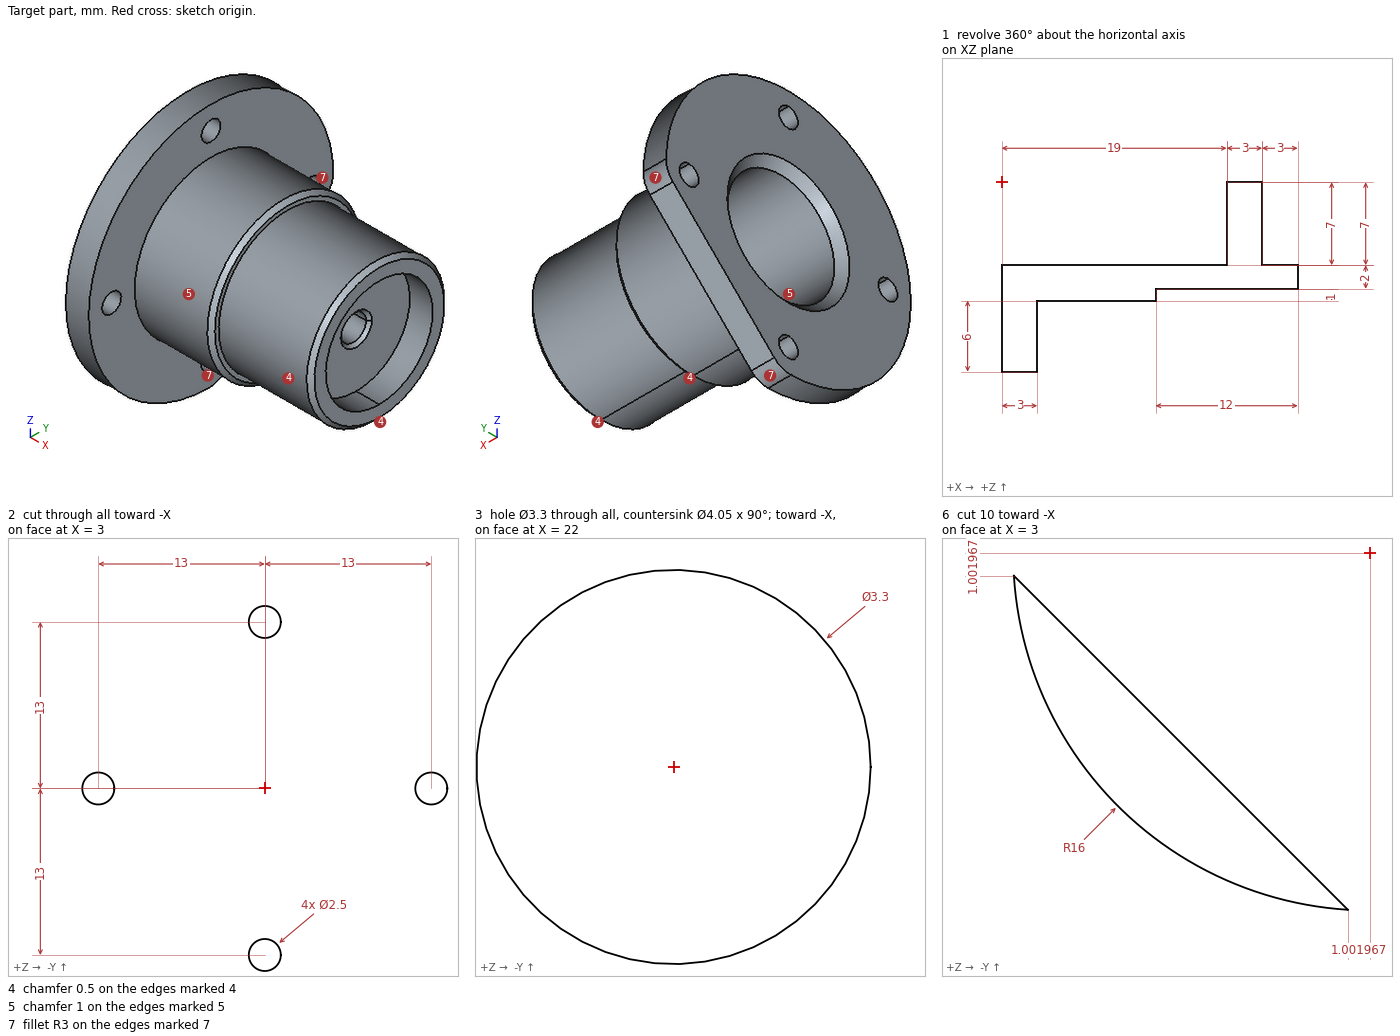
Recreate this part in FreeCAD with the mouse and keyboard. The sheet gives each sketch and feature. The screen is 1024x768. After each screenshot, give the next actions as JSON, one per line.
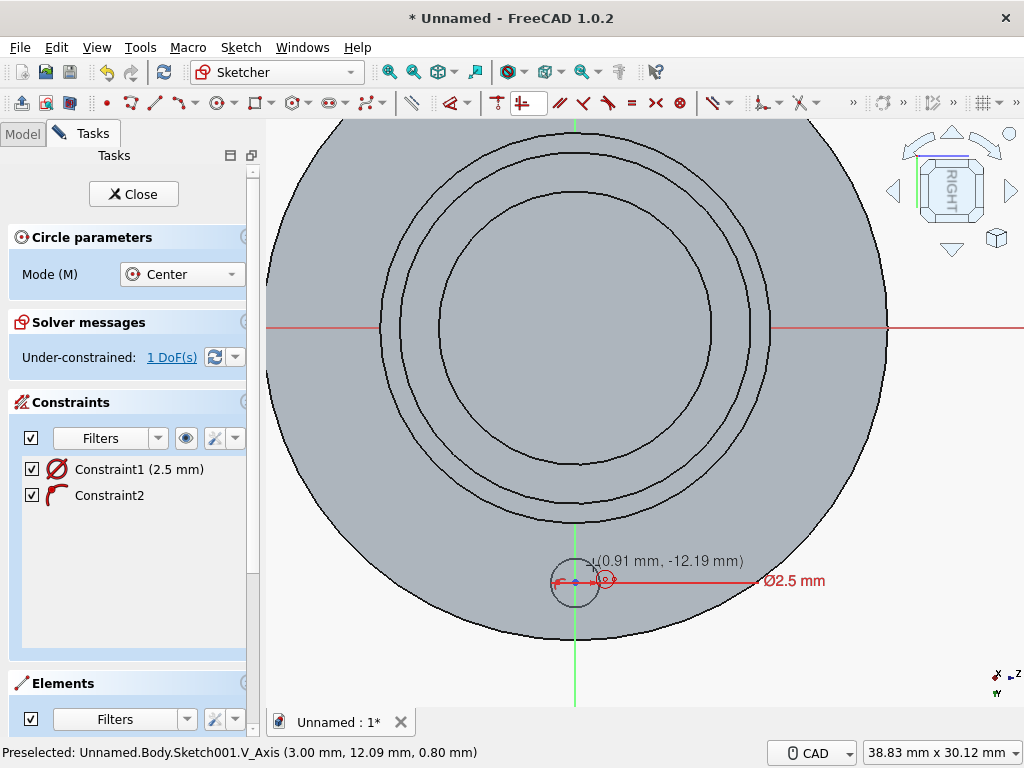
{"action": "left_click", "coordinate": [322, 328]}
{"action": "mouse_move", "coordinate": [339, 311]}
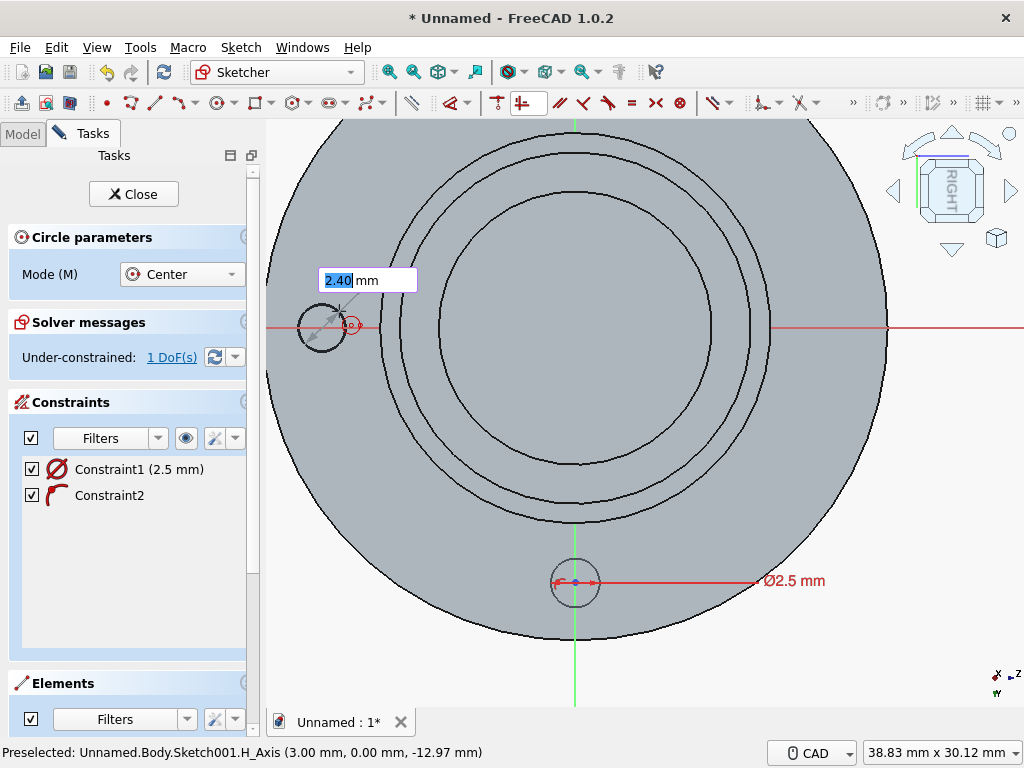
{"action": "type", "text": "2.5"}
{"action": "key", "text": "Return"}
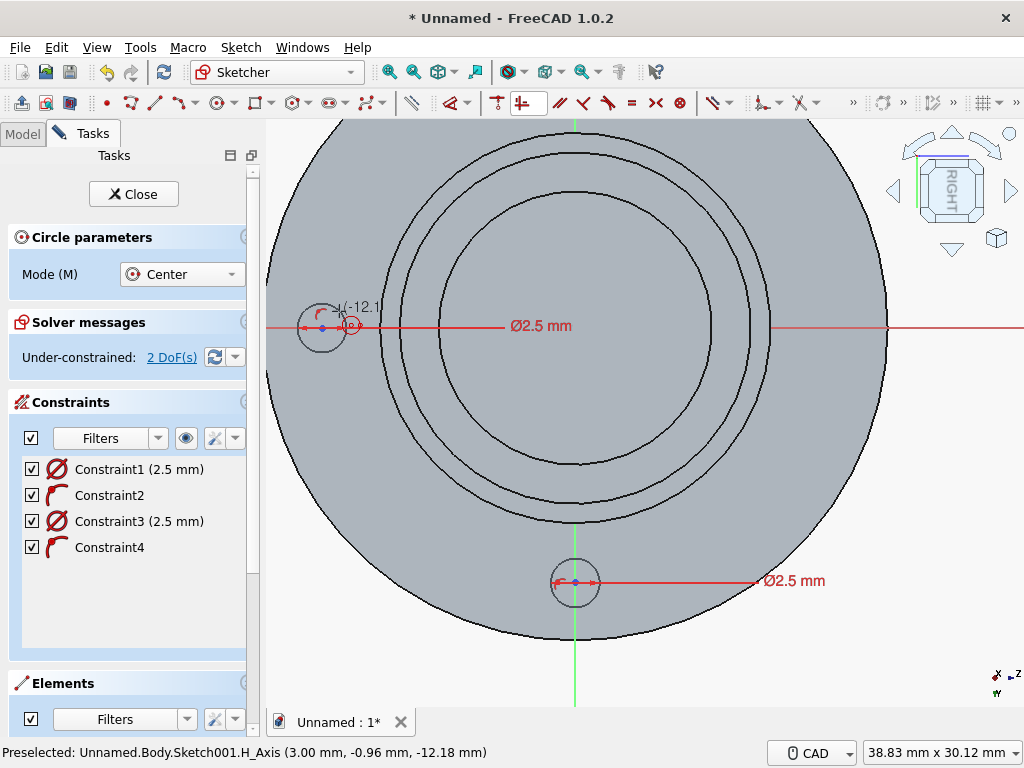
{"action": "scroll", "coordinate": [579, 586], "scroll_direction": "down", "scroll_amount": 2}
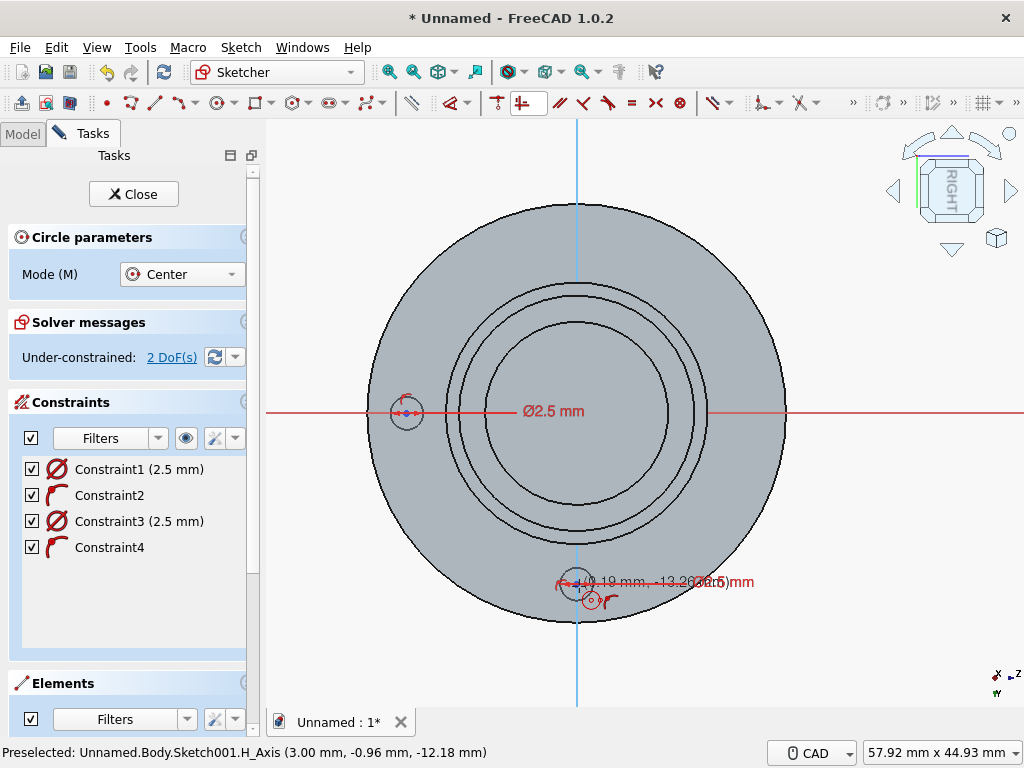
{"action": "scroll", "coordinate": [577, 243], "scroll_direction": "up", "scroll_amount": 2}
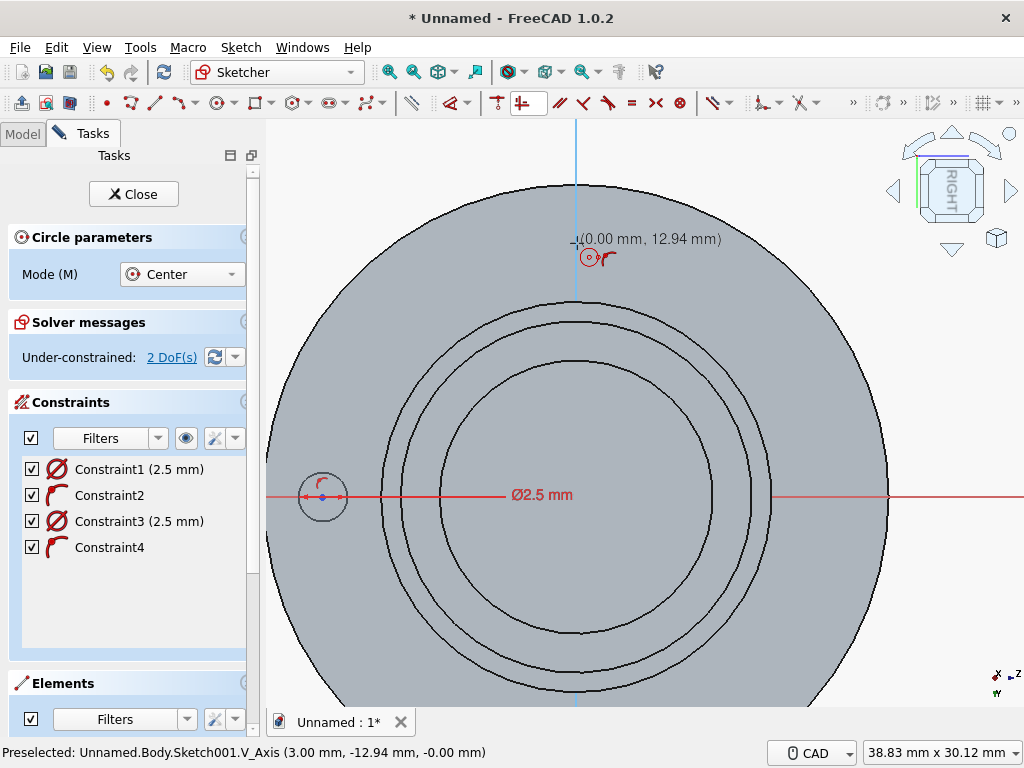
{"action": "left_click", "coordinate": [576, 243]}
{"action": "mouse_move", "coordinate": [594, 226]}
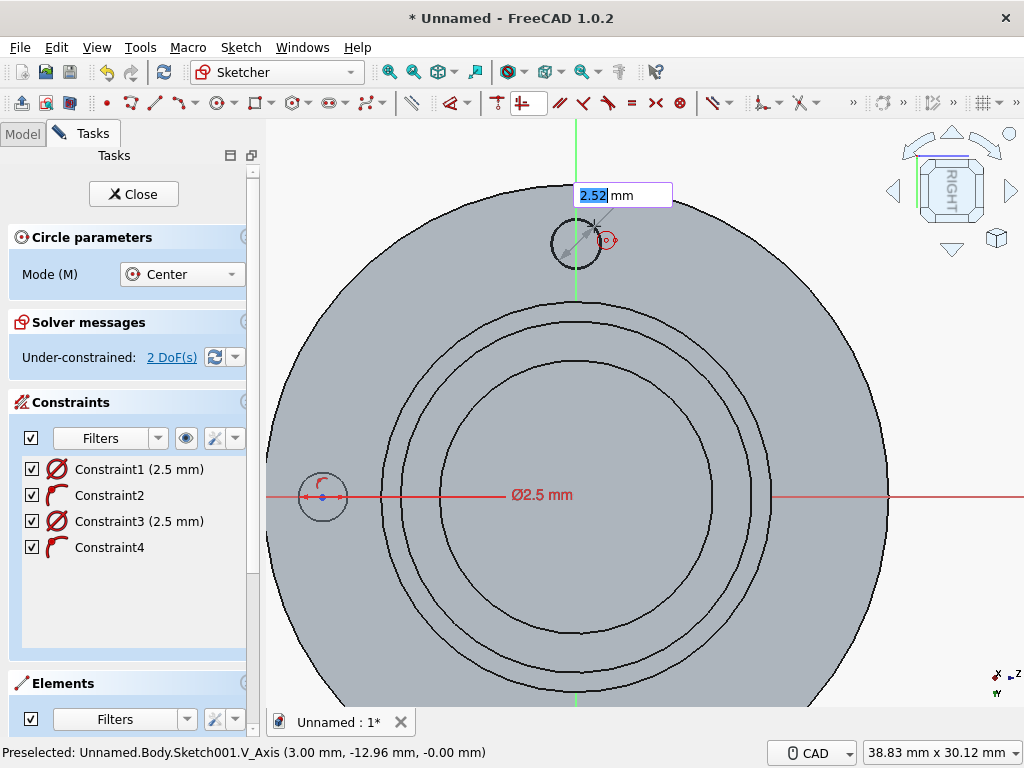
{"action": "type", "text": "2.5"}
{"action": "key", "text": "Return"}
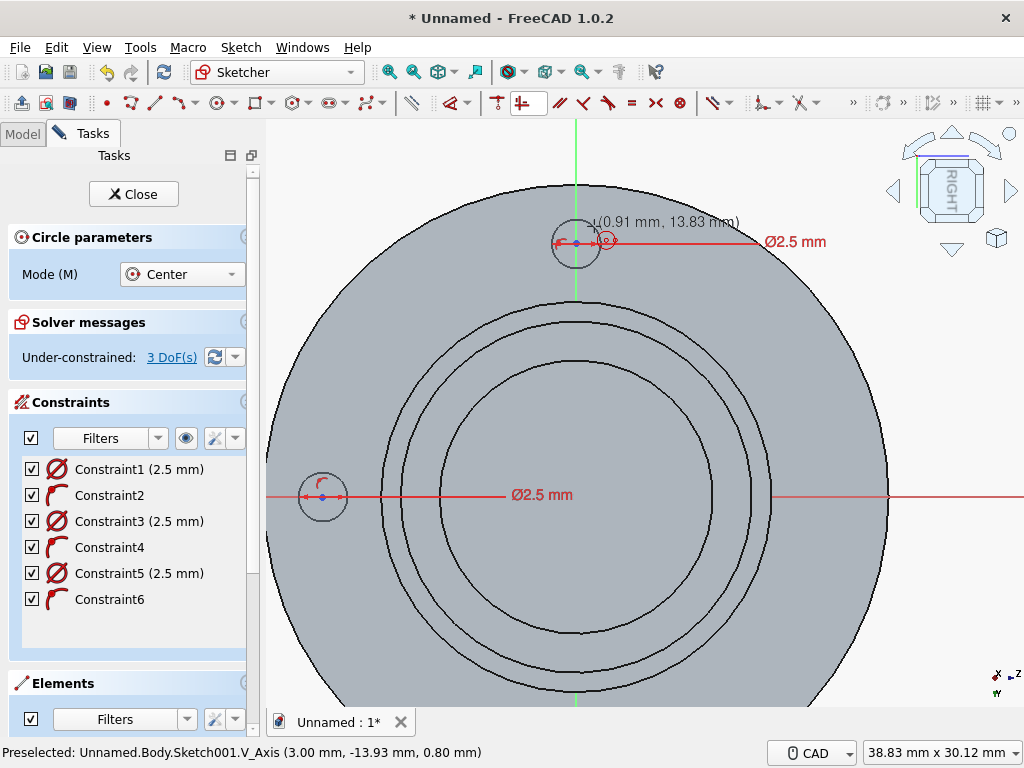
{"action": "left_click", "coordinate": [830, 497]}
{"action": "mouse_move", "coordinate": [847, 480]}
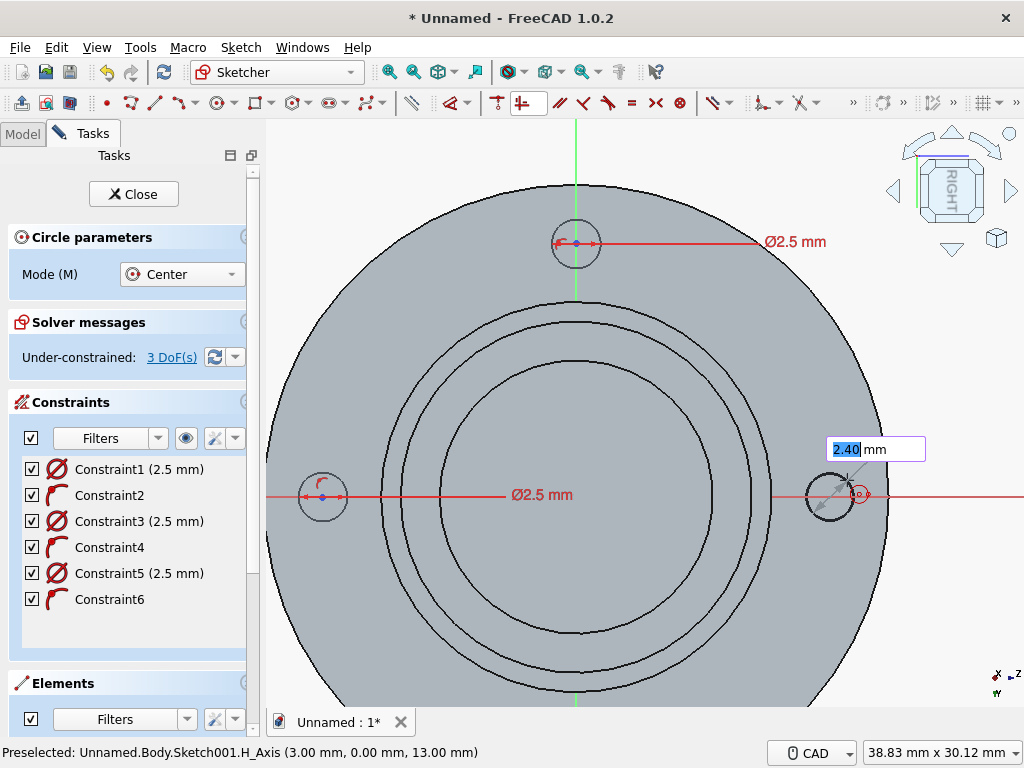
{"action": "type", "text": "2.5"}
{"action": "key", "text": "Return"}
{"action": "key", "text": "Escape"}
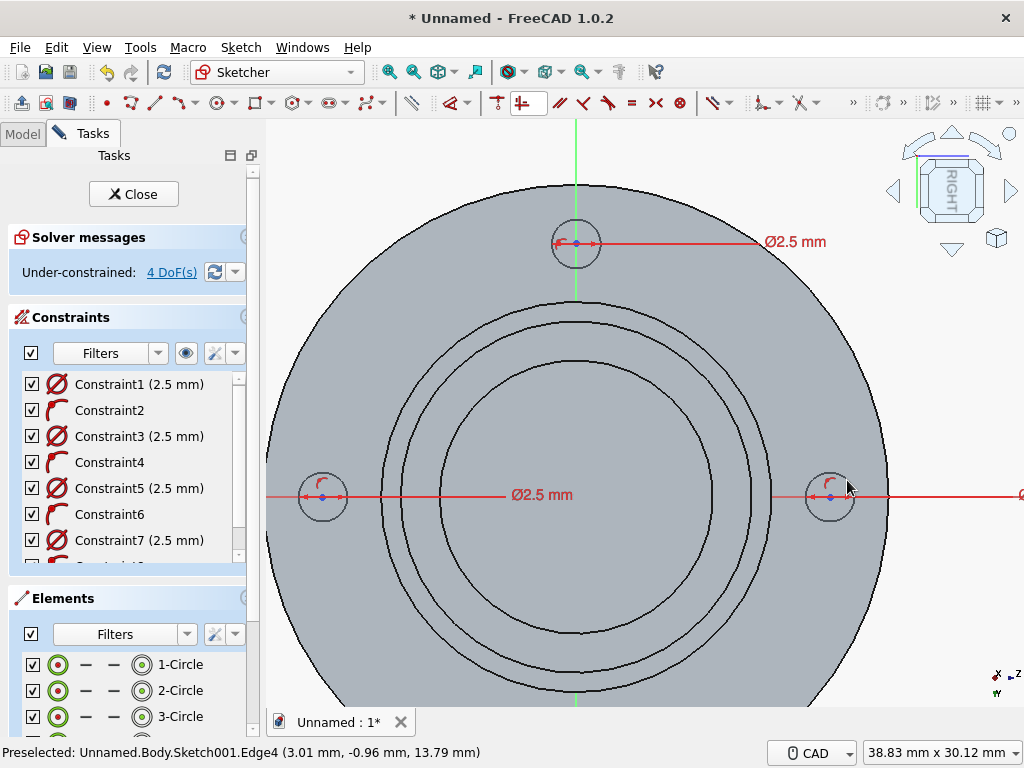
{"action": "left_click", "coordinate": [450, 104]}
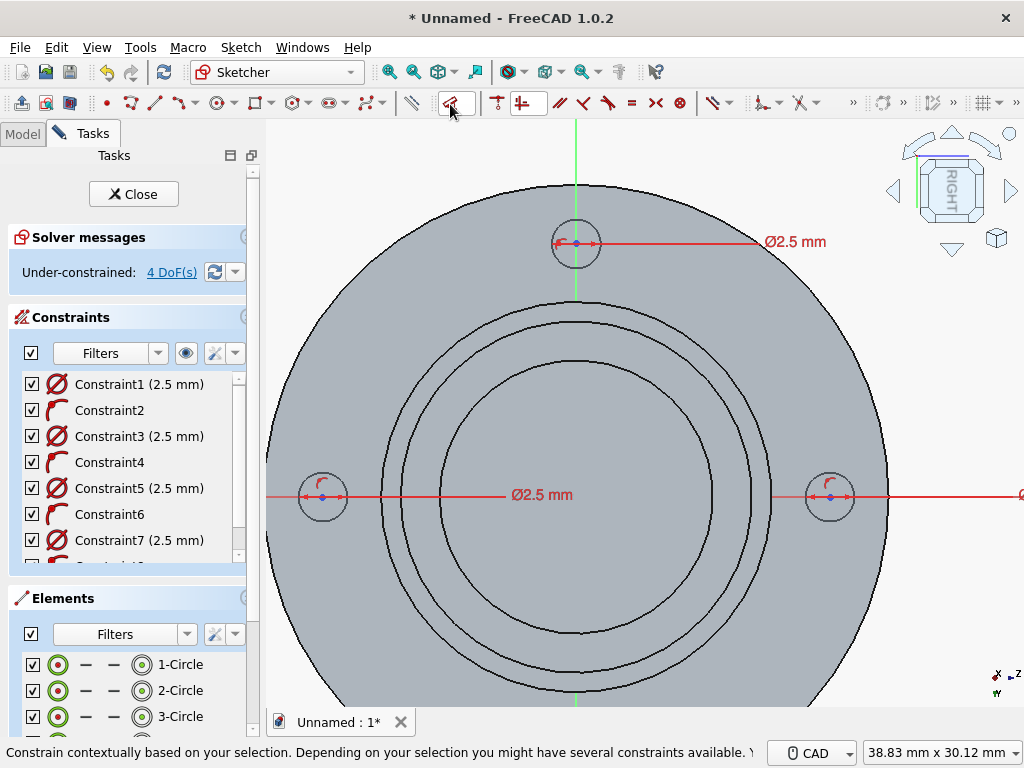
{"action": "scroll", "coordinate": [577, 242], "scroll_direction": "down", "scroll_amount": 2}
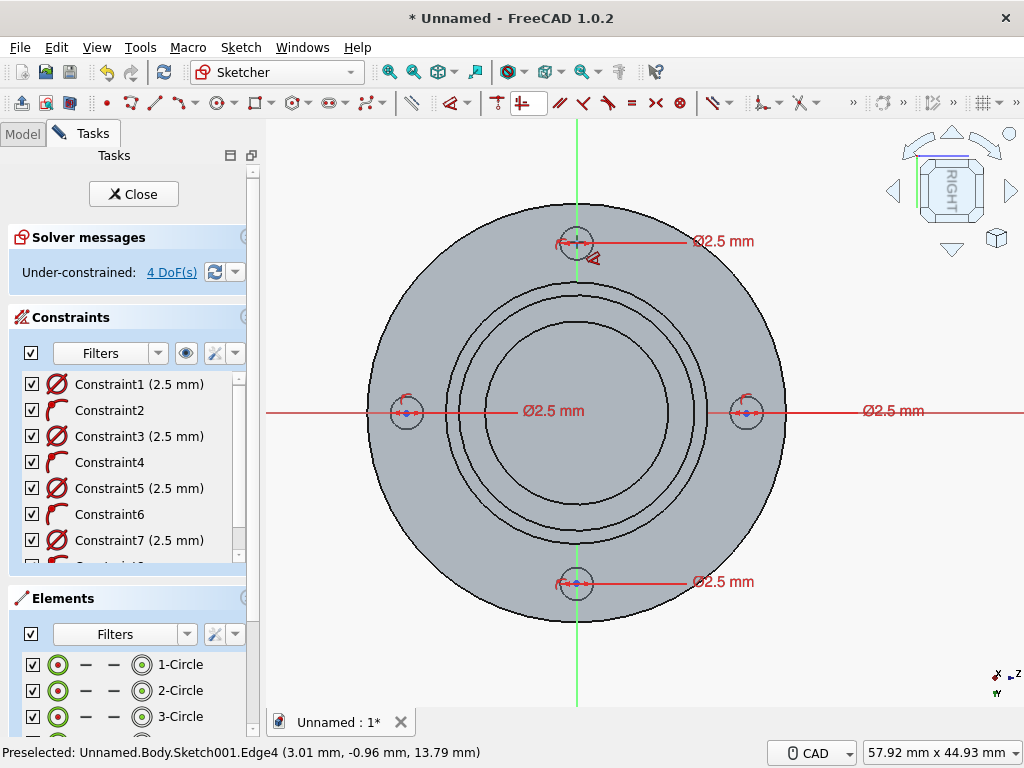
{"action": "left_click", "coordinate": [577, 584]}
{"action": "left_click", "coordinate": [611, 498]}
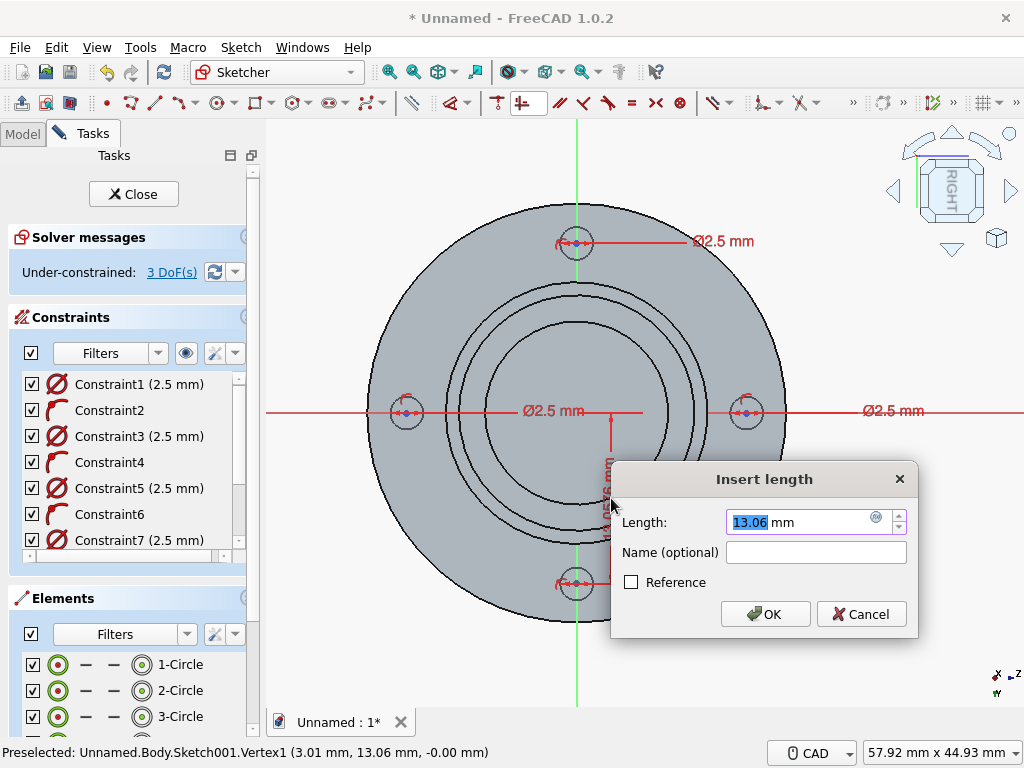
{"action": "type", "text": "13"}
{"action": "key", "text": "Return"}